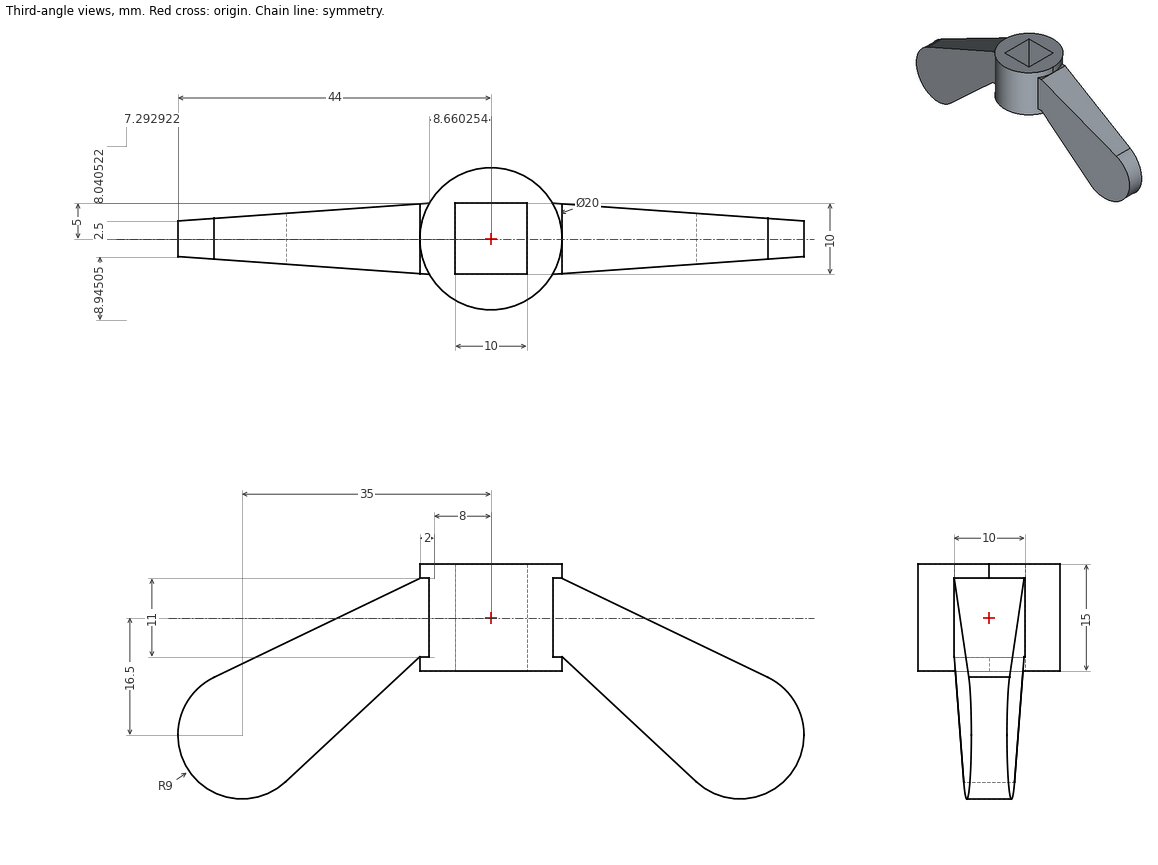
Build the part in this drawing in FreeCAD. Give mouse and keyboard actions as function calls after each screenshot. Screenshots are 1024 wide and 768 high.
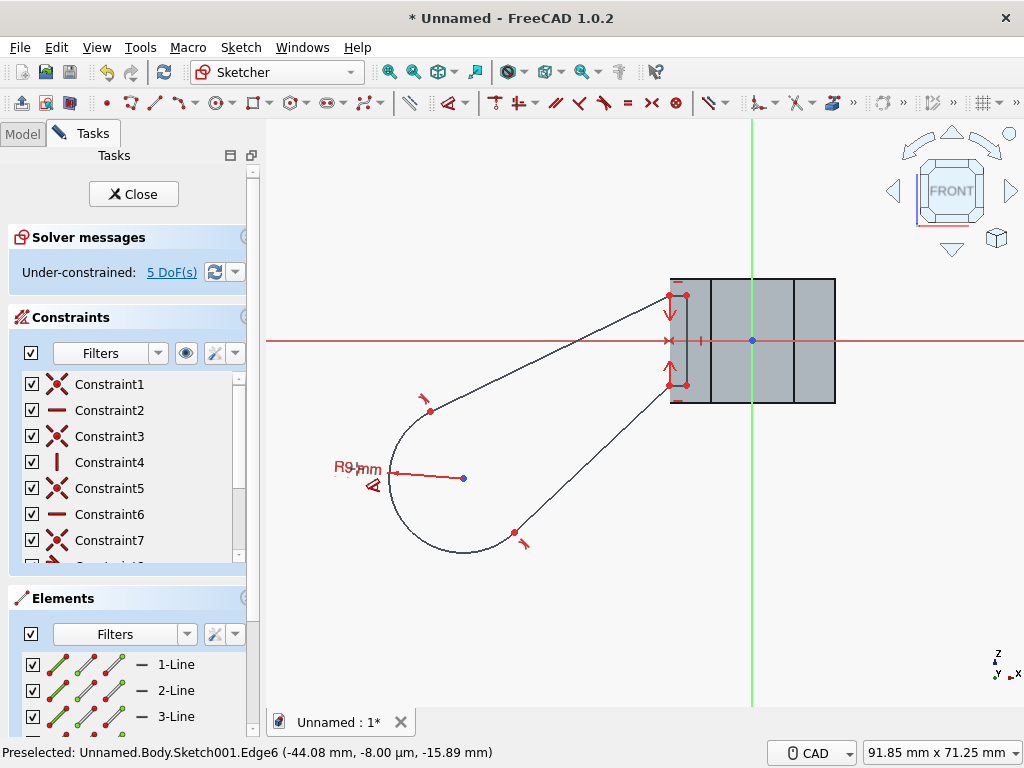
scroll(678, 296, up, 5)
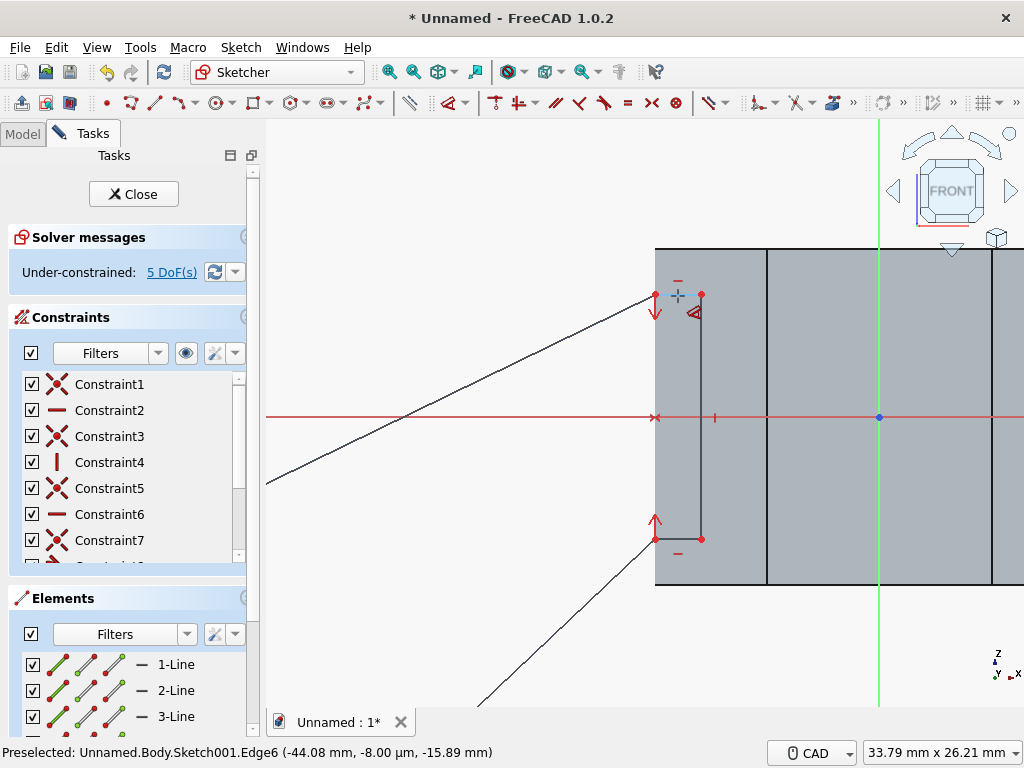
click(678, 295)
click(678, 261)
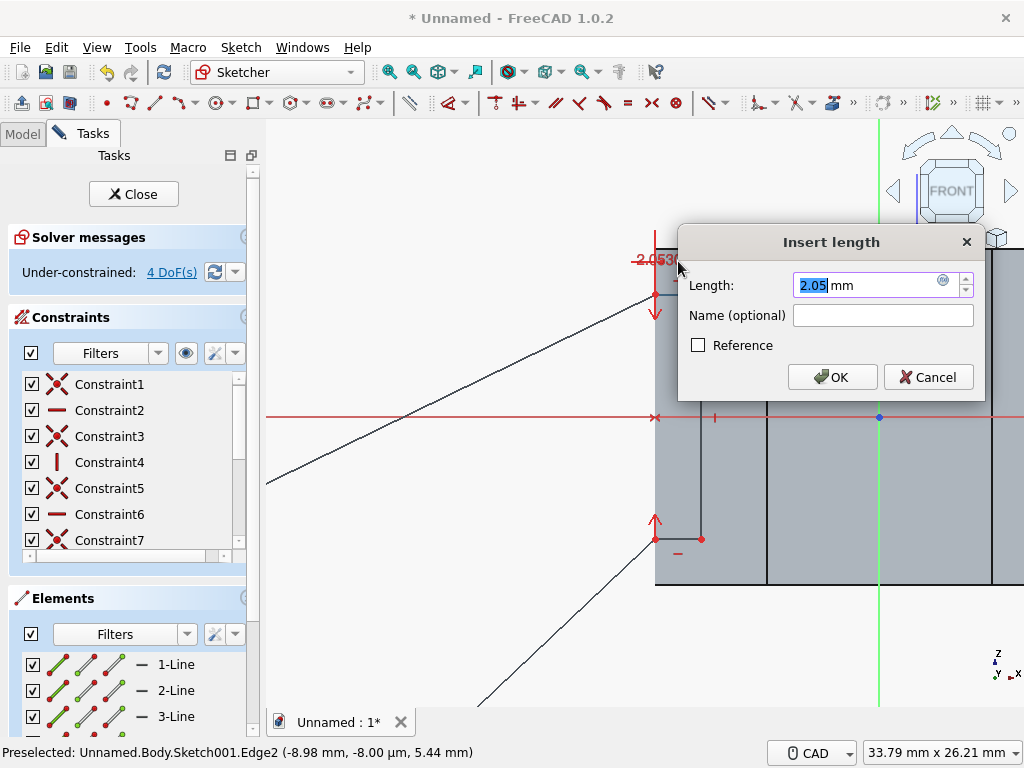
text(2)
key(Return)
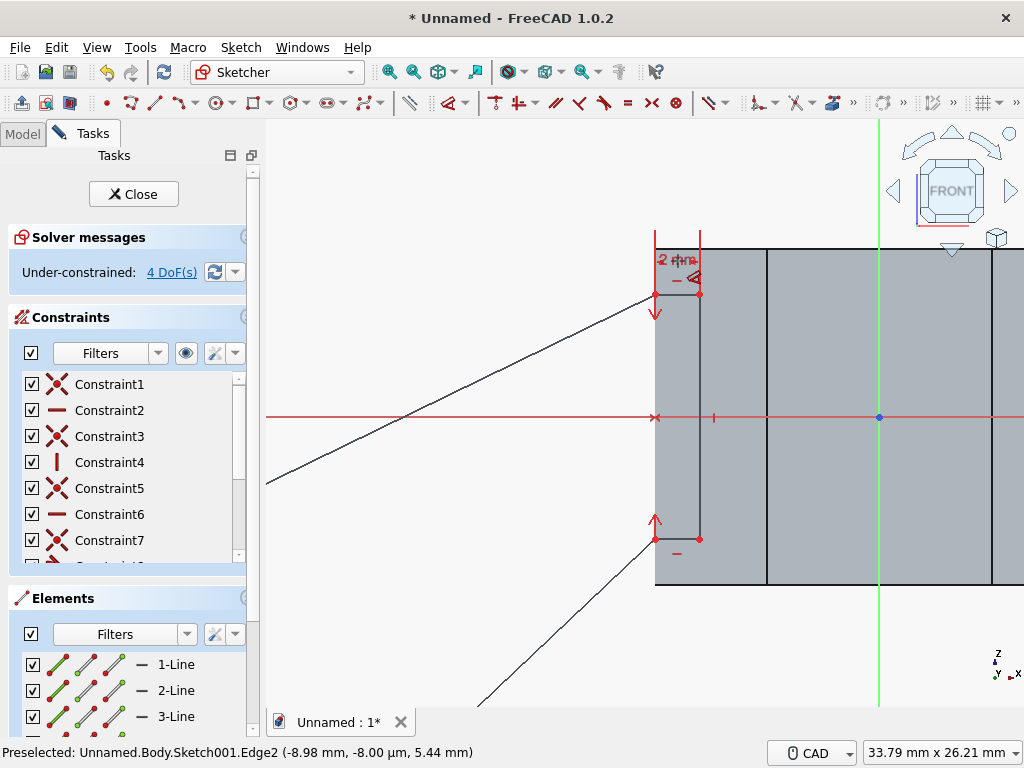
click(700, 368)
click(734, 361)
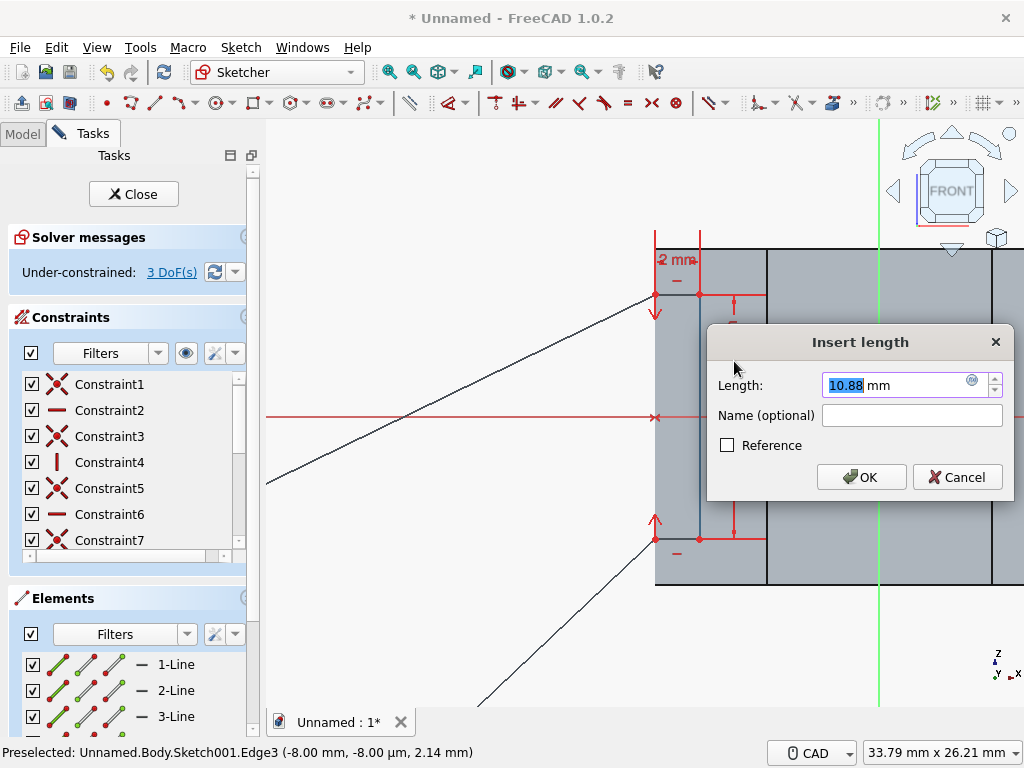
text(11)
key(Return)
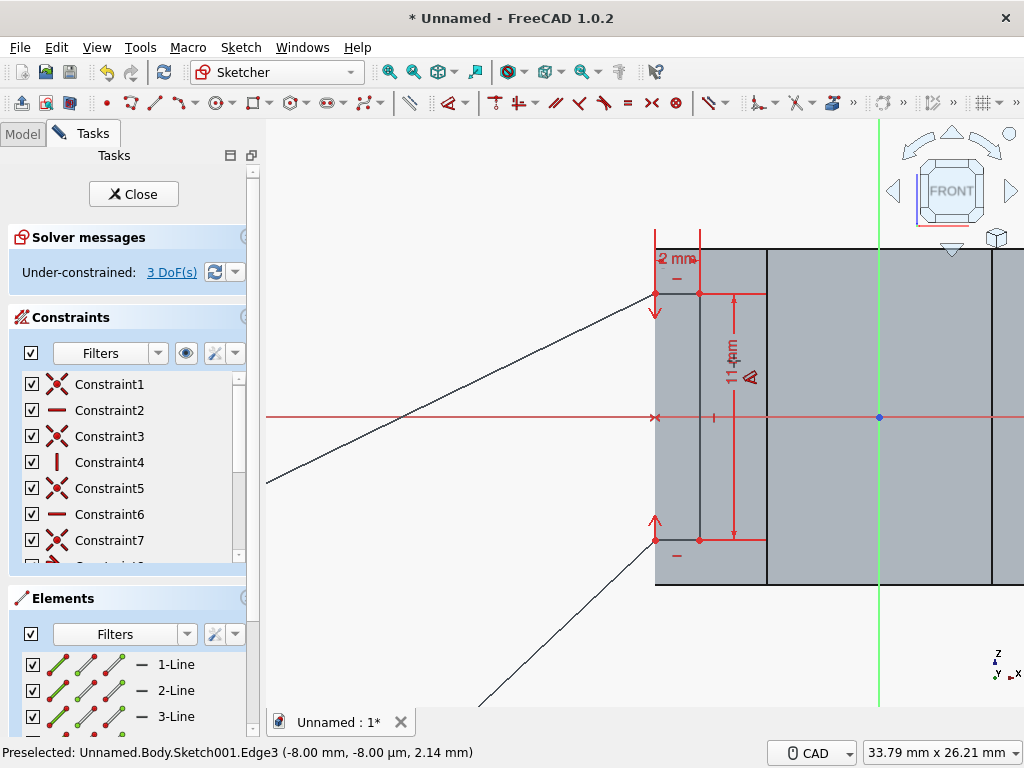
click(700, 294)
click(779, 260)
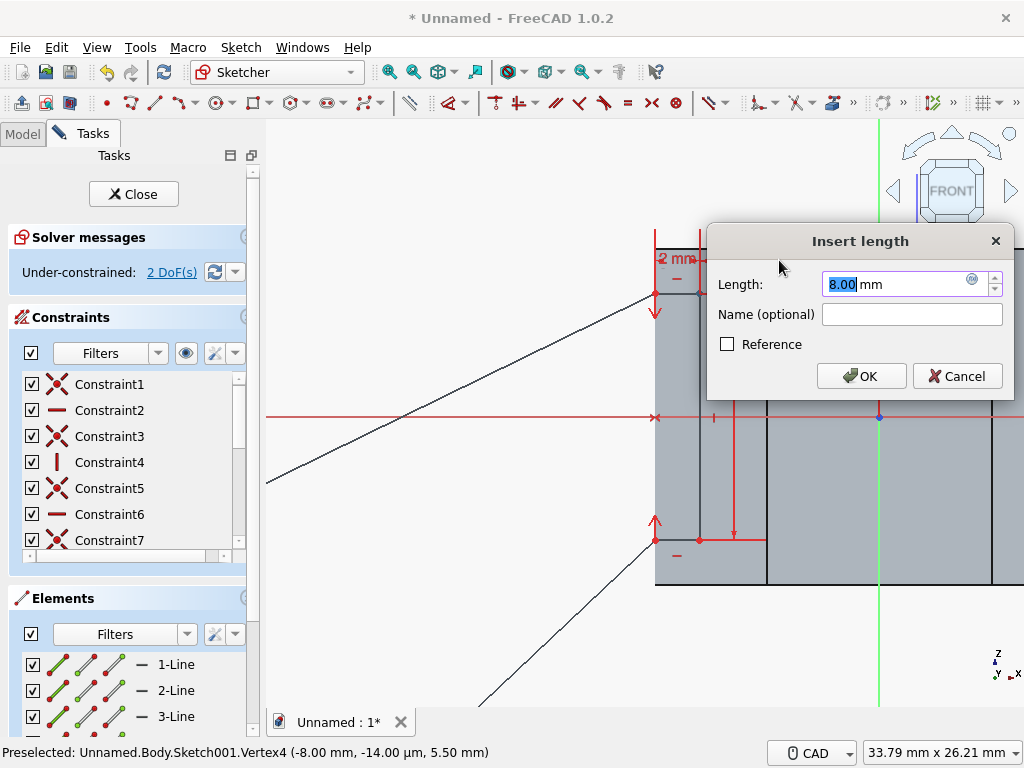
text(8)
key(Return)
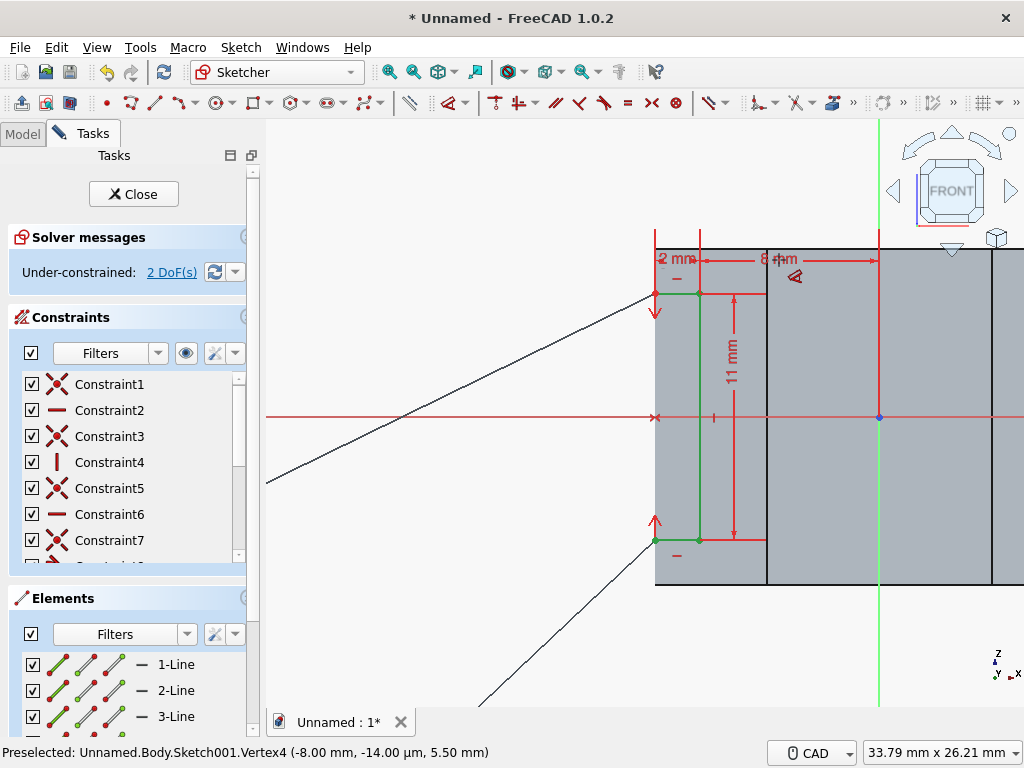
scroll(718, 249, down, 4)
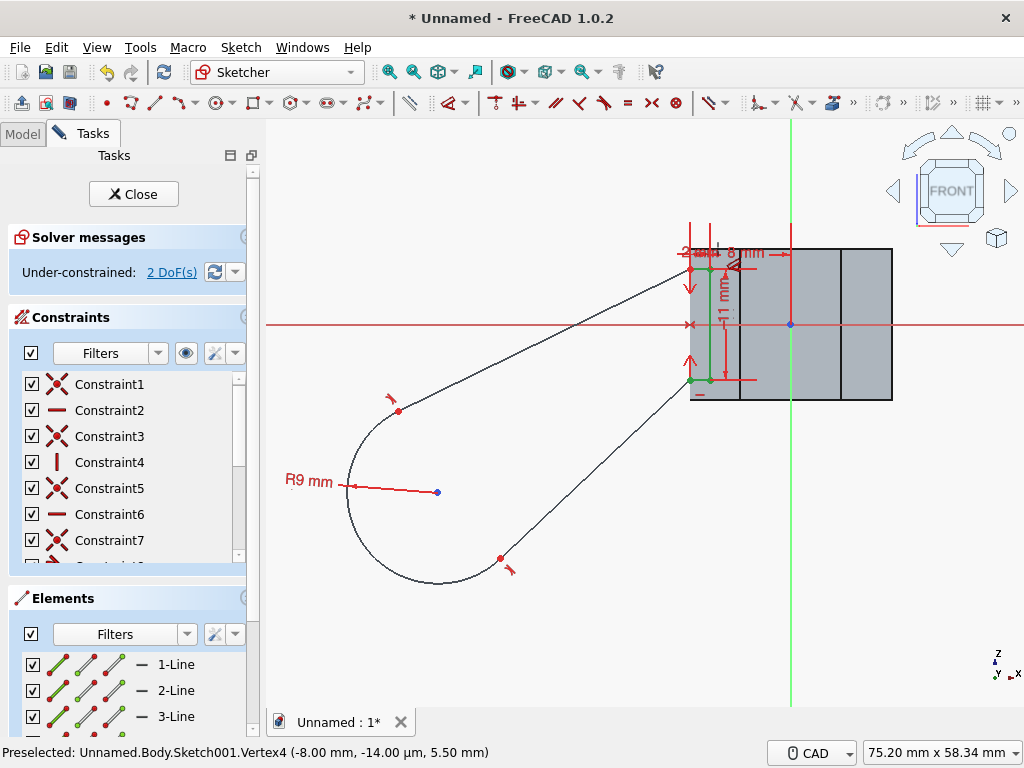
click(438, 493)
click(614, 291)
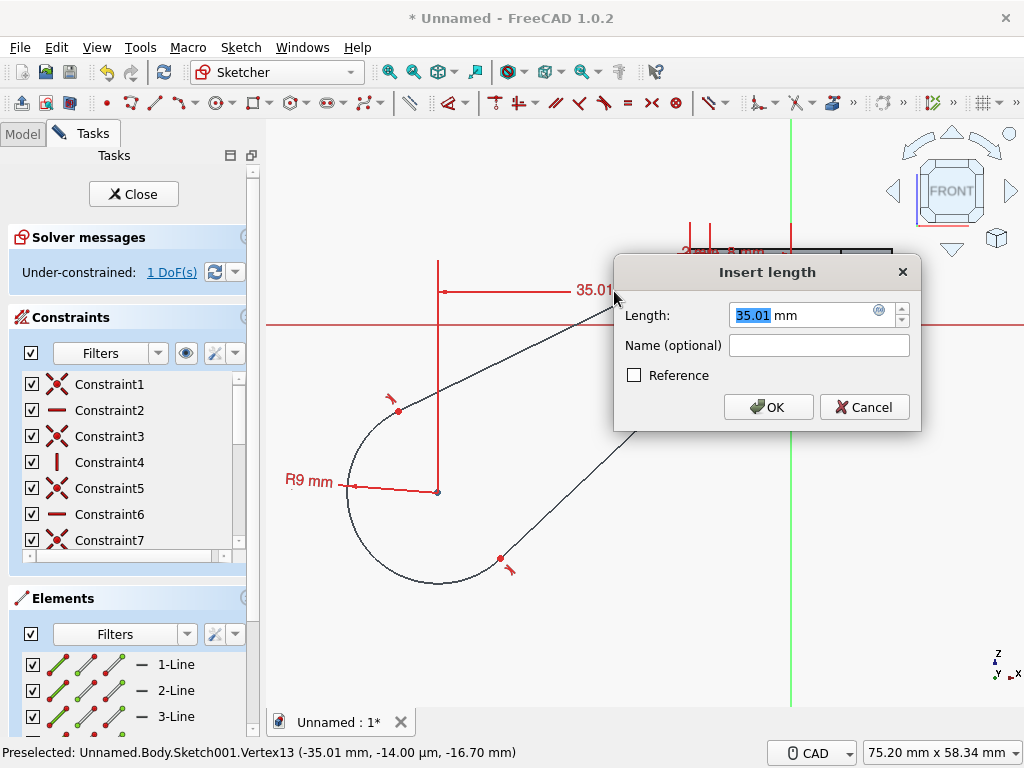
text(35)
key(Return)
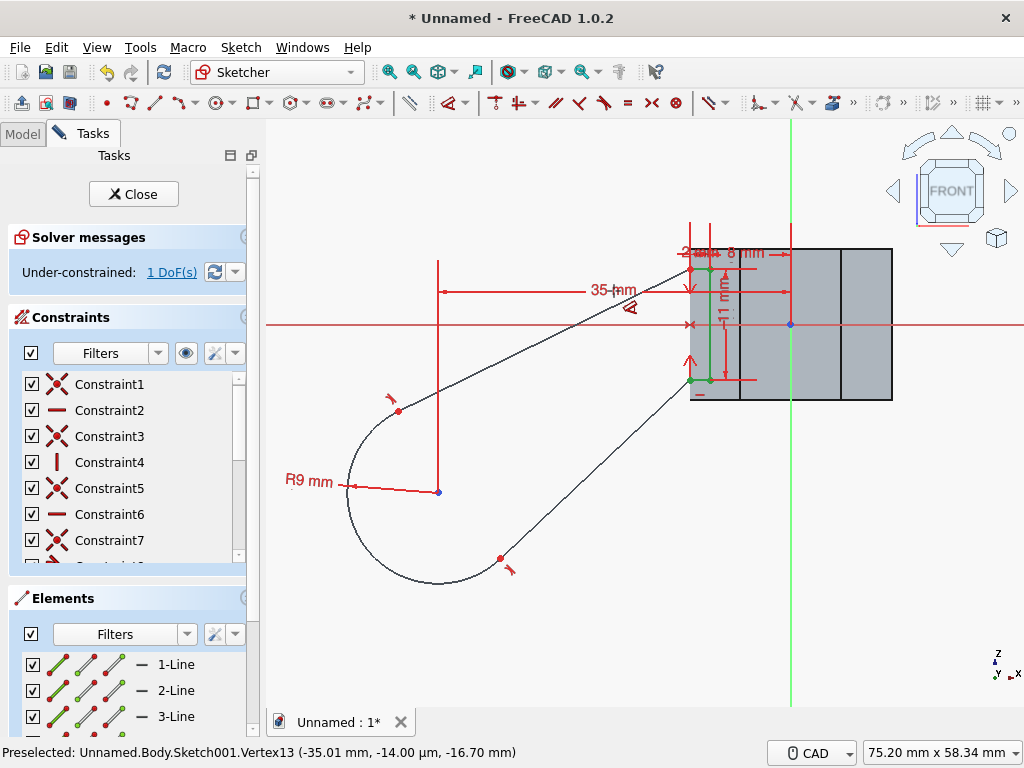
click(438, 493)
click(825, 409)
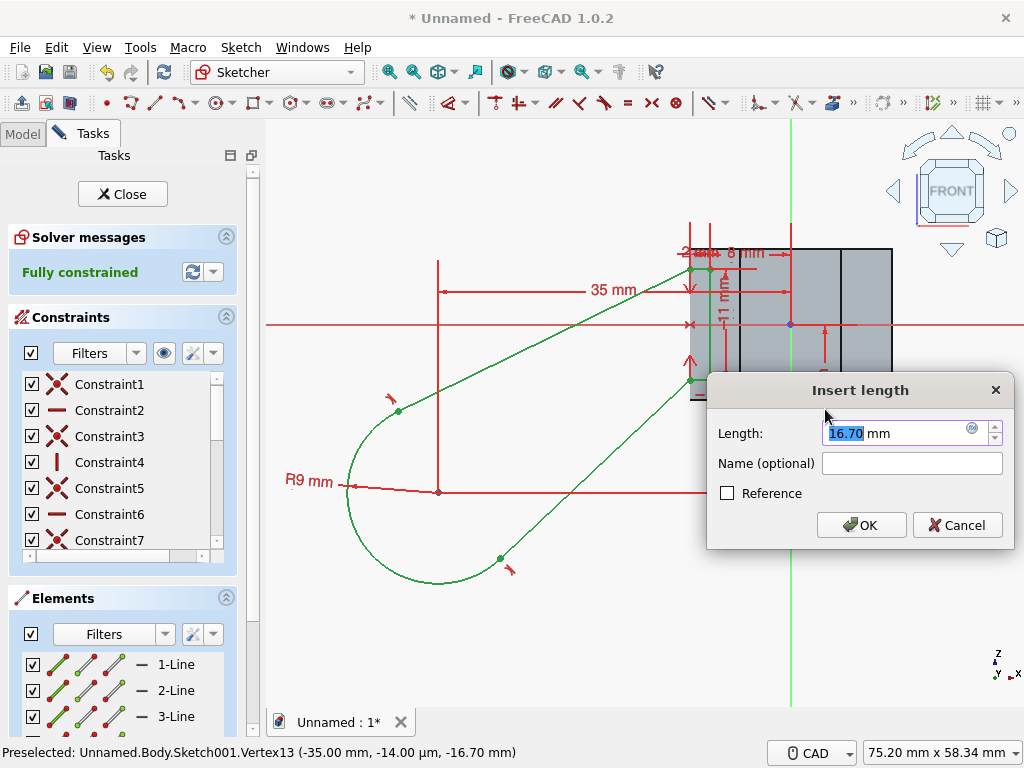
text(16.5)
key(Return)
key(Escape)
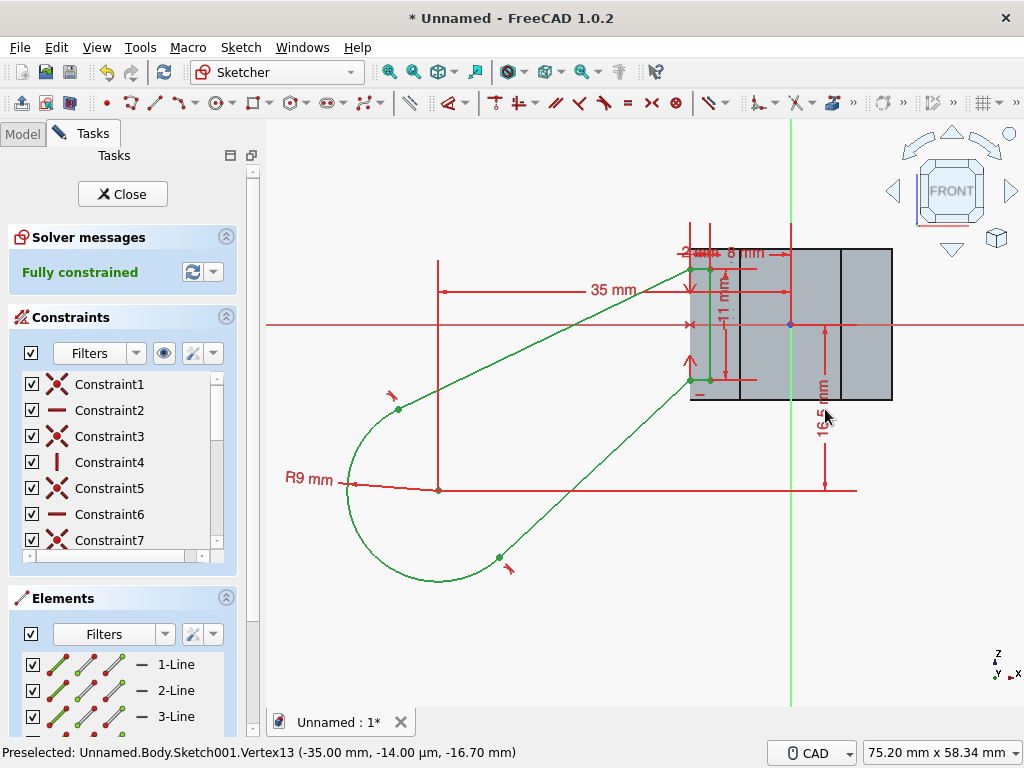
click(123, 194)